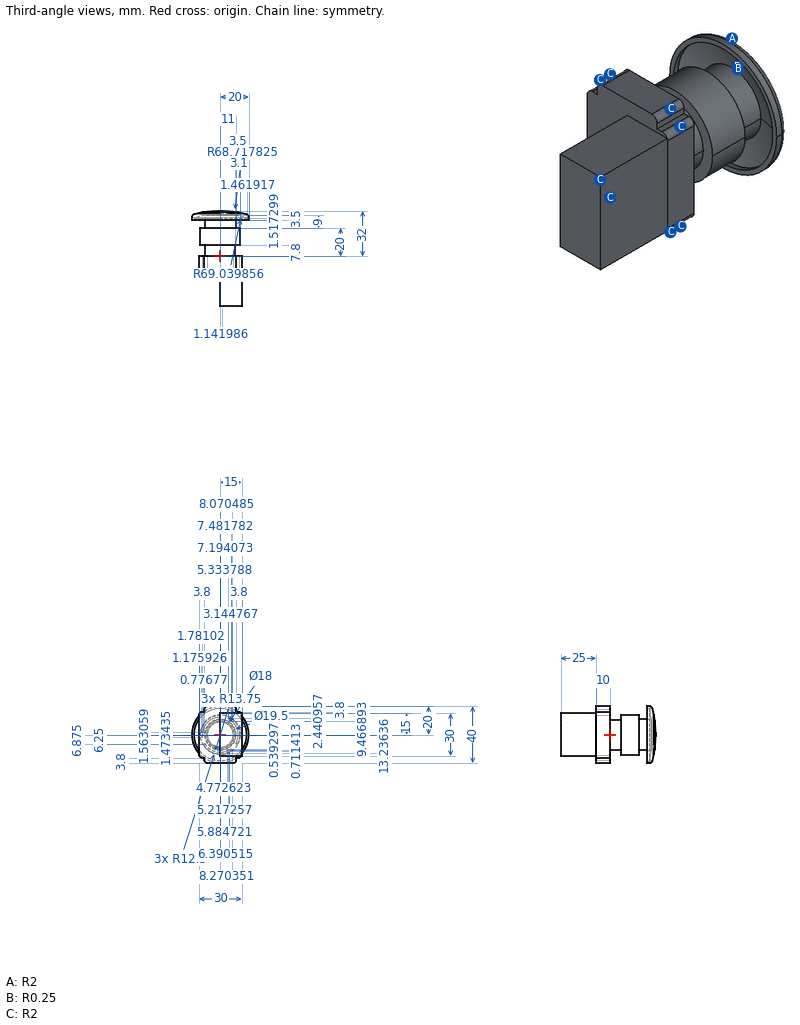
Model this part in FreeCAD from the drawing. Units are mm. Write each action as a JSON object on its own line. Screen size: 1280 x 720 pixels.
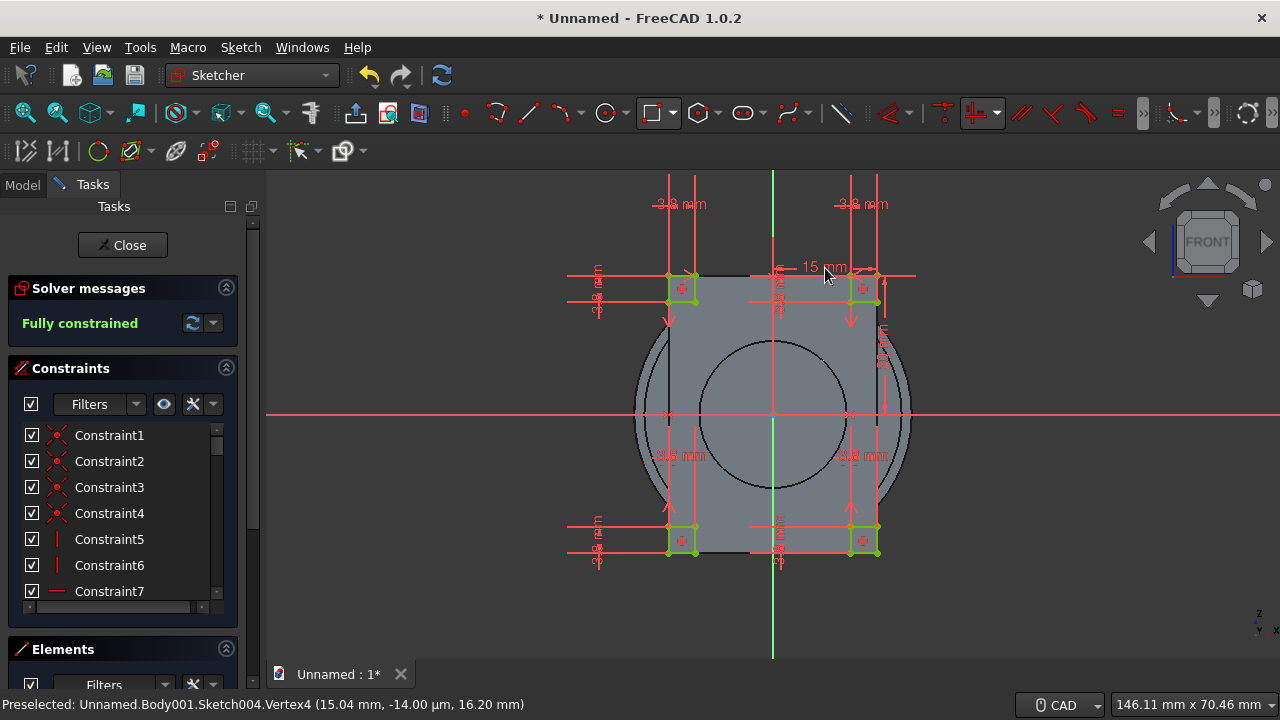
{"action": "left_click", "coordinate": [123, 245]}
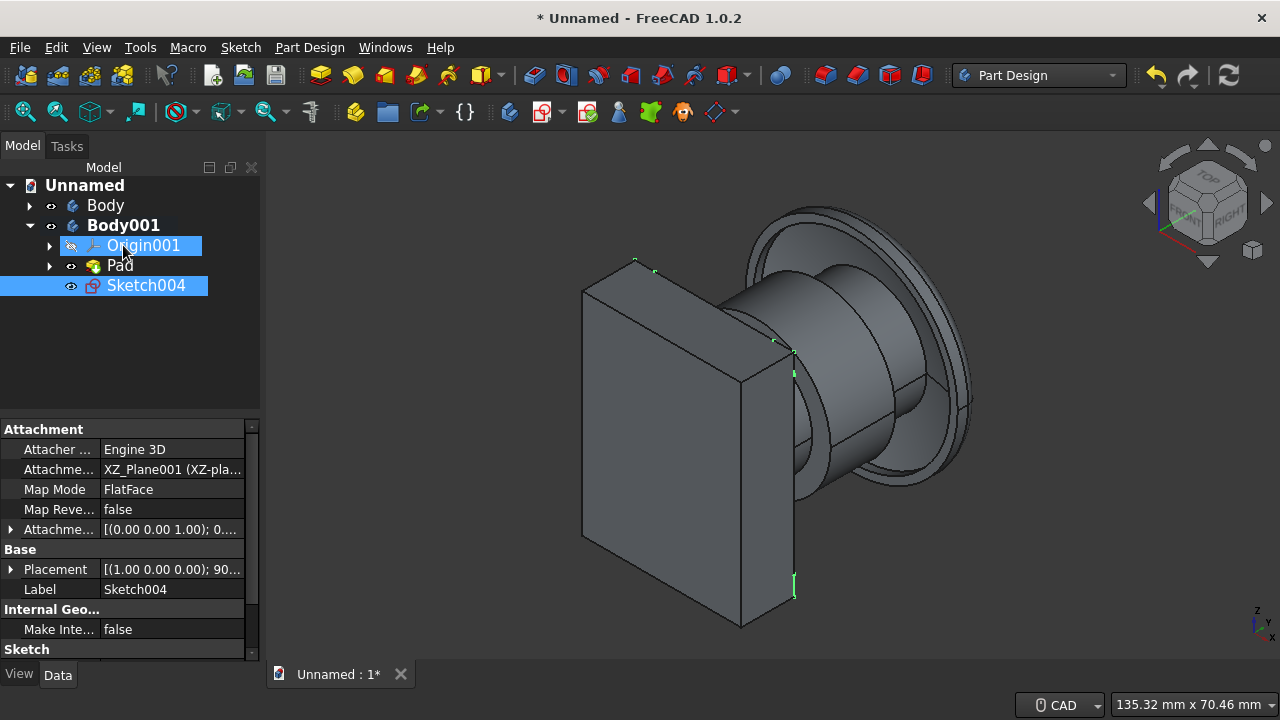
{"action": "left_click", "coordinate": [536, 76]}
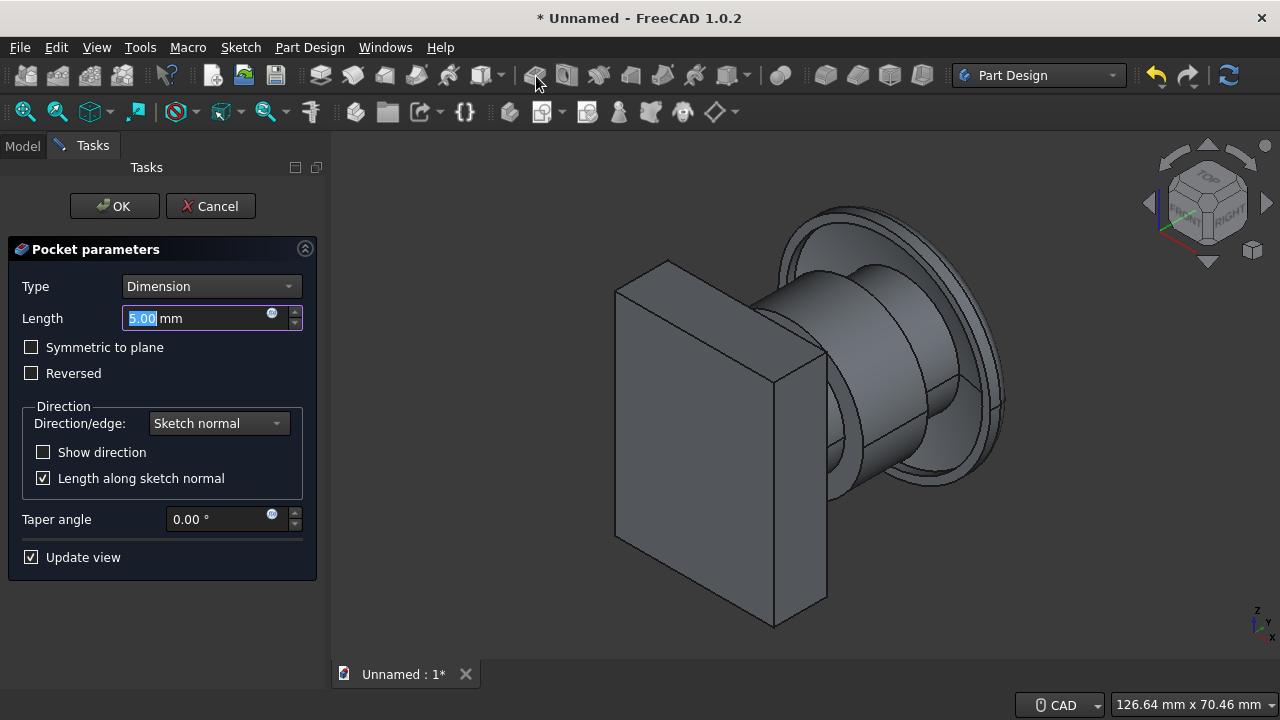
{"action": "type", "text": "10"}
{"action": "key", "text": "Tab"}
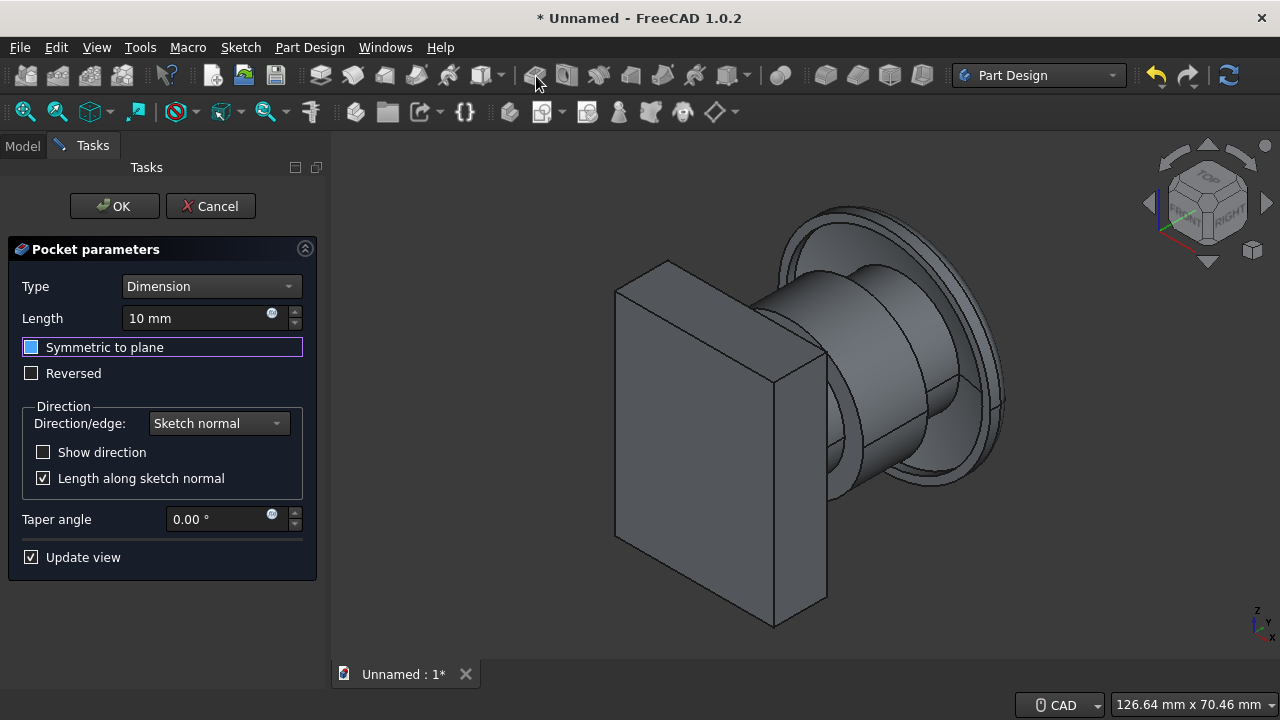
{"action": "left_click", "coordinate": [30, 373]}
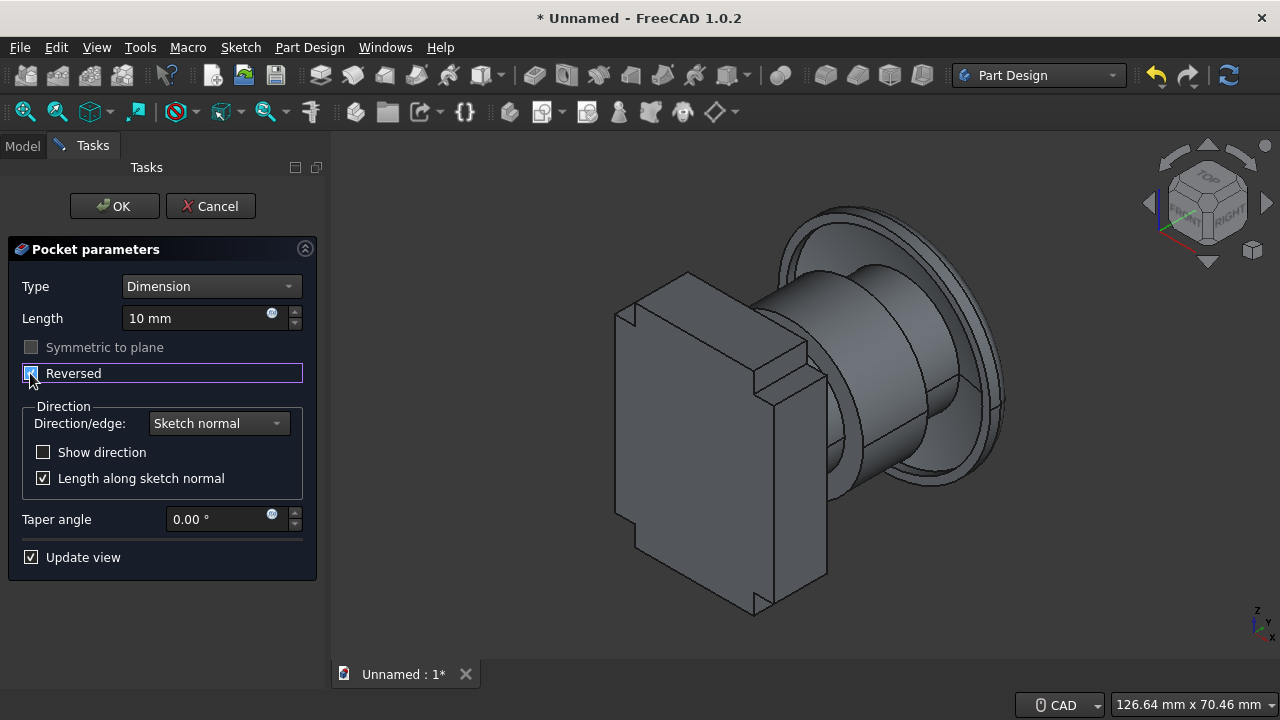
{"action": "left_click", "coordinate": [115, 206]}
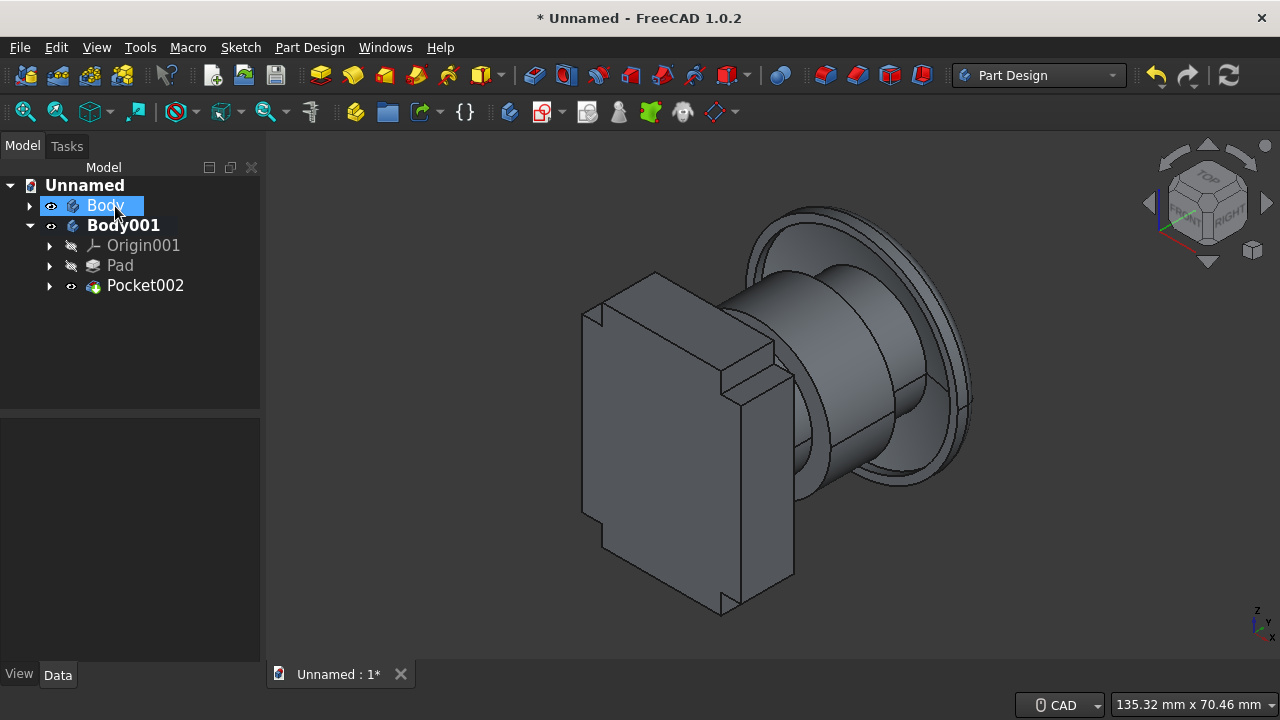
{"action": "left_click", "coordinate": [768, 390]}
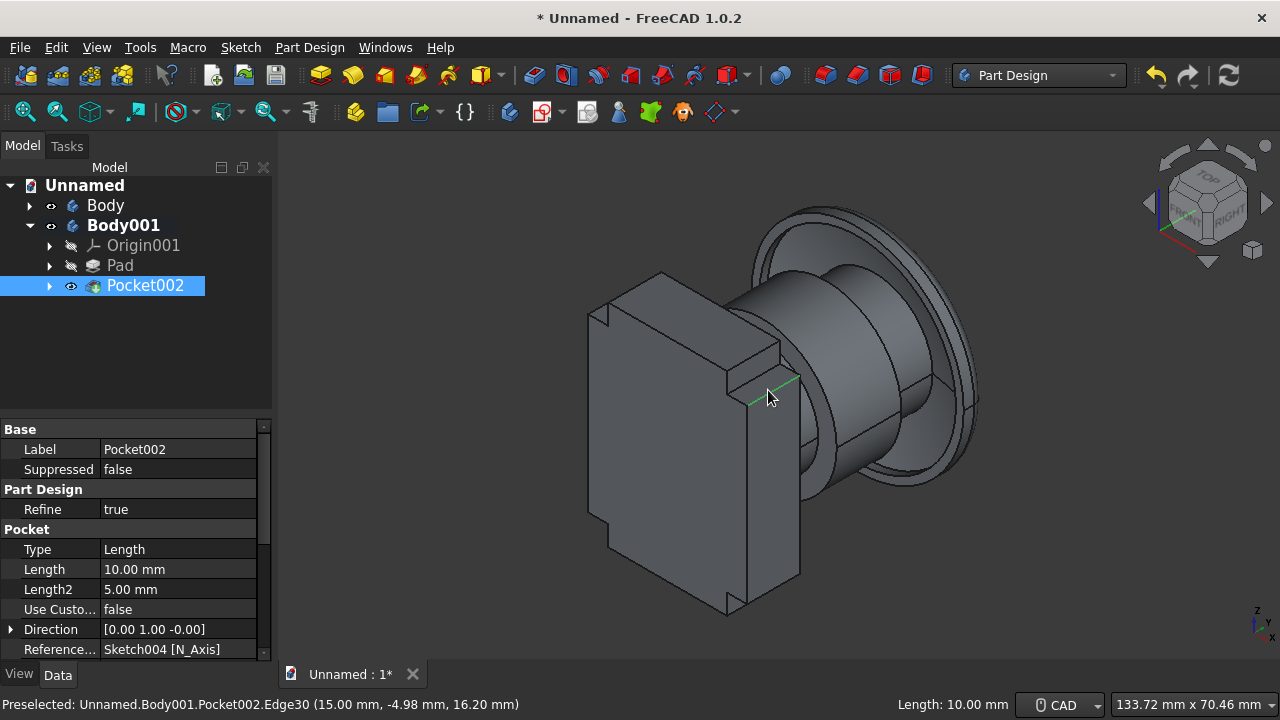
{"action": "left_click", "coordinate": [754, 355], "text": "ctrl"}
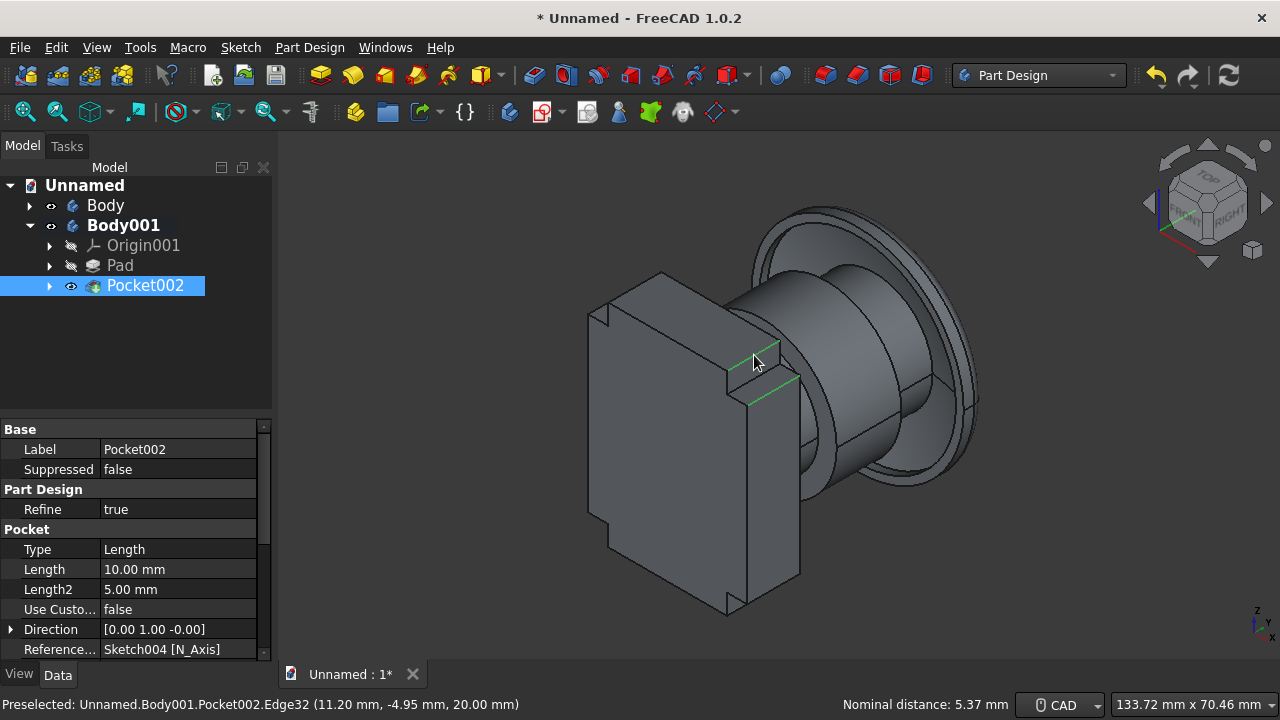
{"action": "key", "text": "2"}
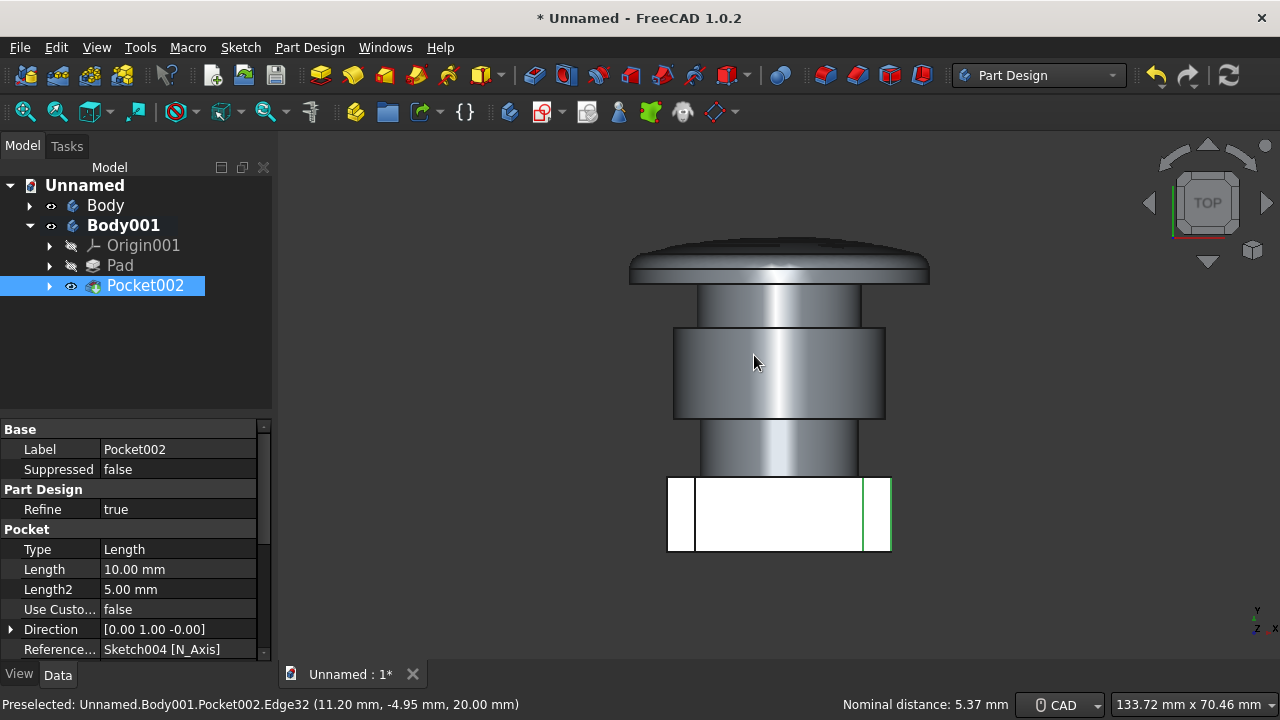
{"action": "left_click", "coordinate": [26, 112]}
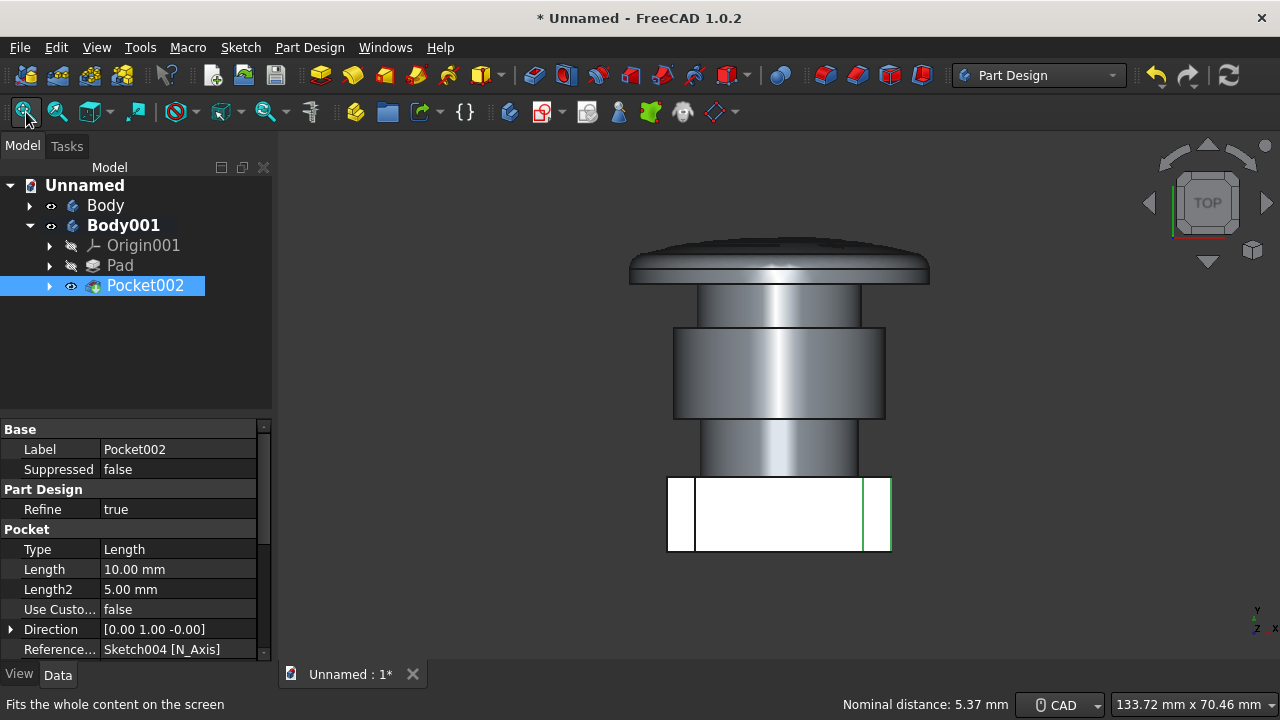
{"action": "left_click", "coordinate": [695, 514], "text": "ctrl"}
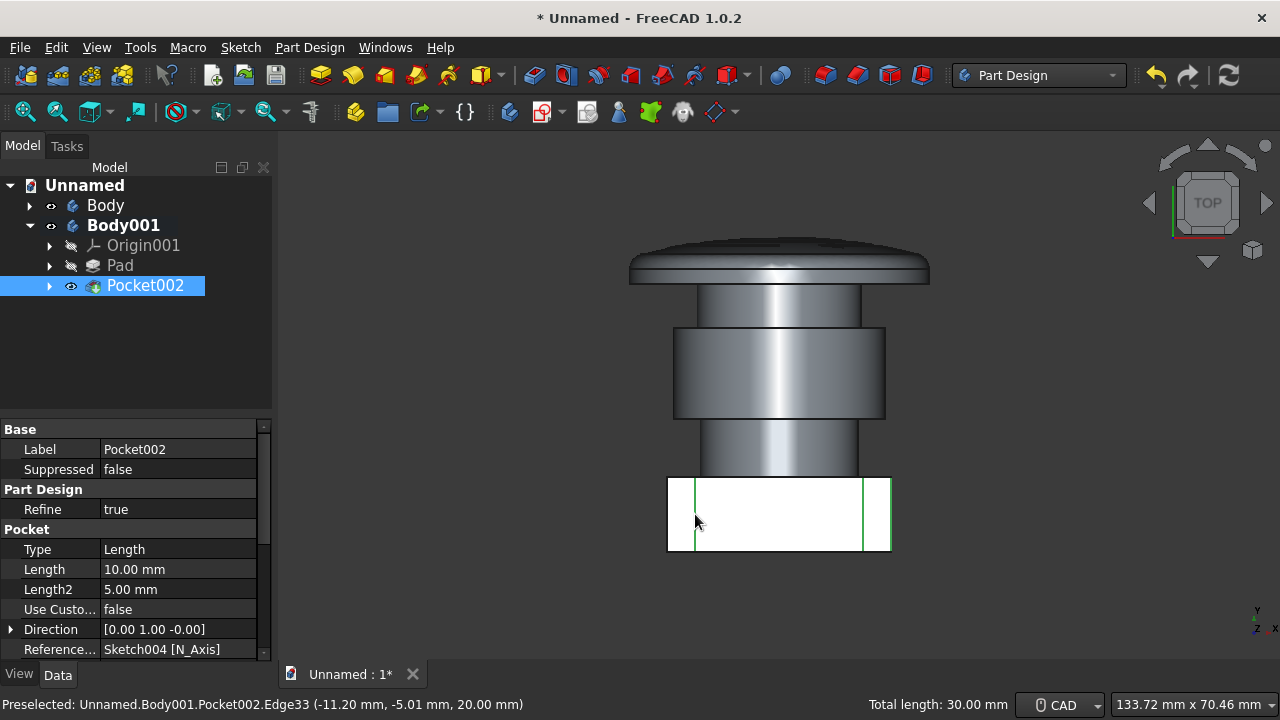
{"action": "left_click", "coordinate": [667, 514], "text": "ctrl"}